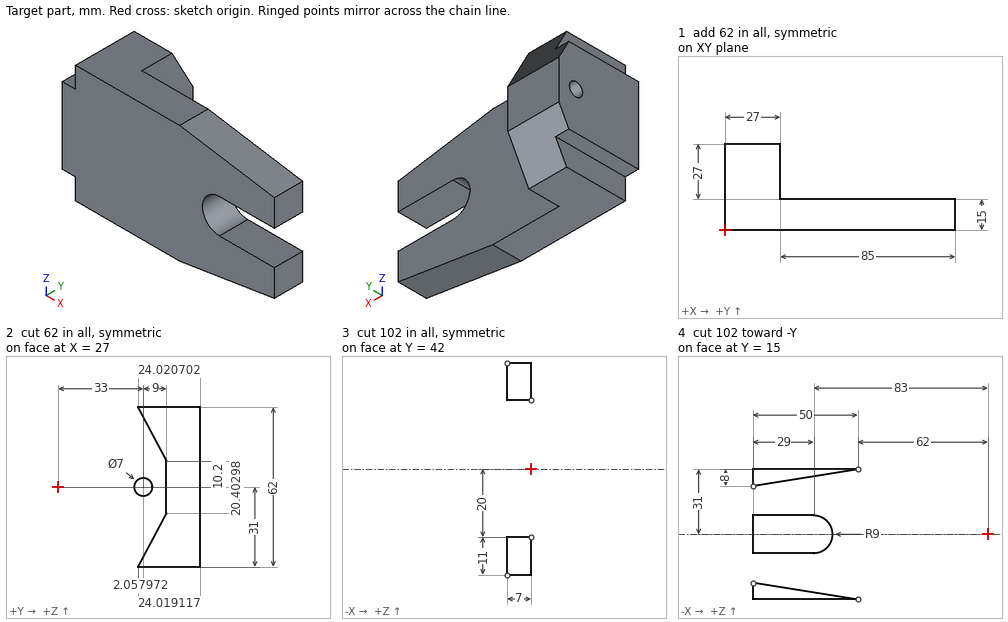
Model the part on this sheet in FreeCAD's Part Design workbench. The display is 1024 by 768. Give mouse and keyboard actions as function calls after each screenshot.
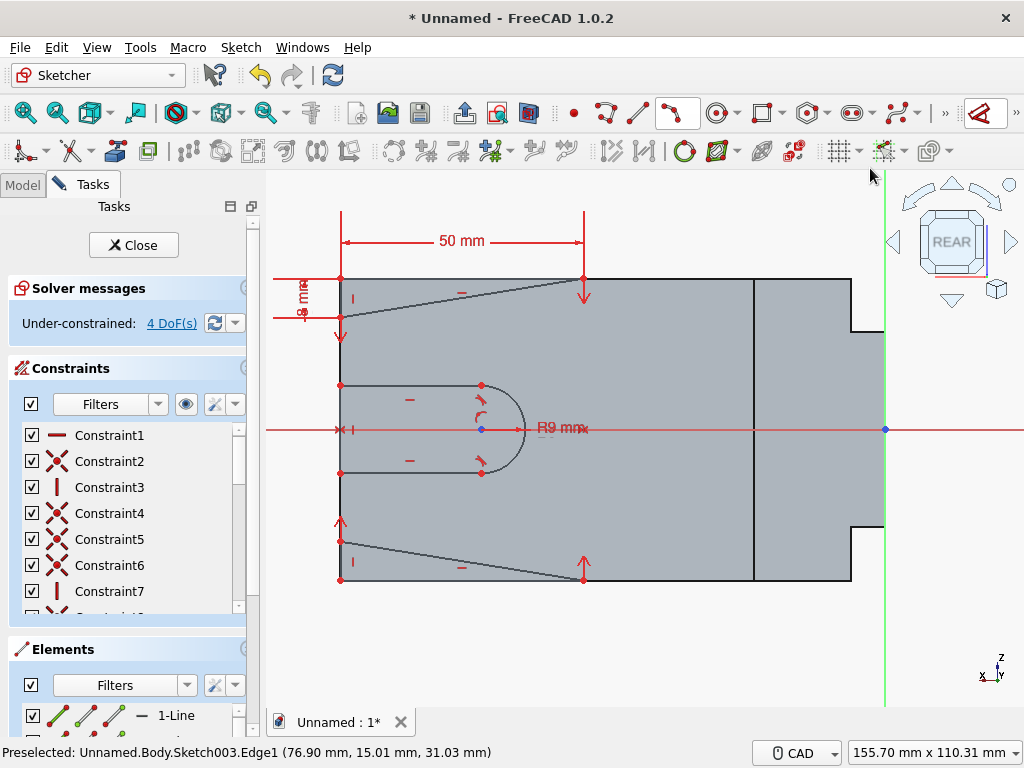
click(439, 386)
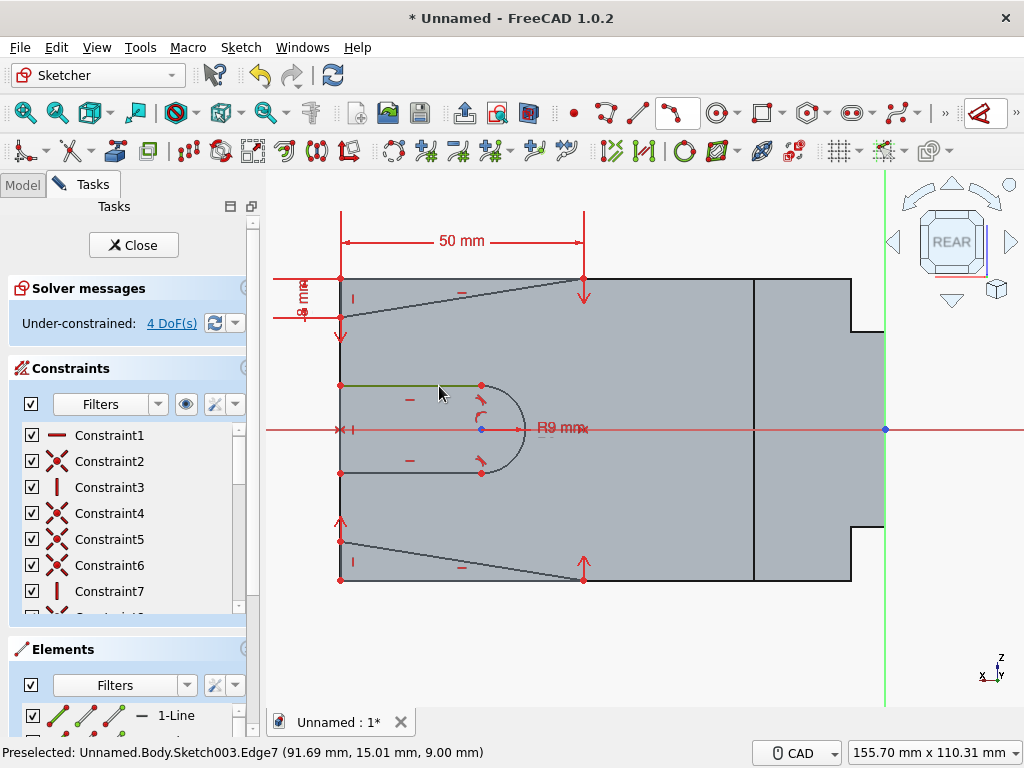
click(1002, 114)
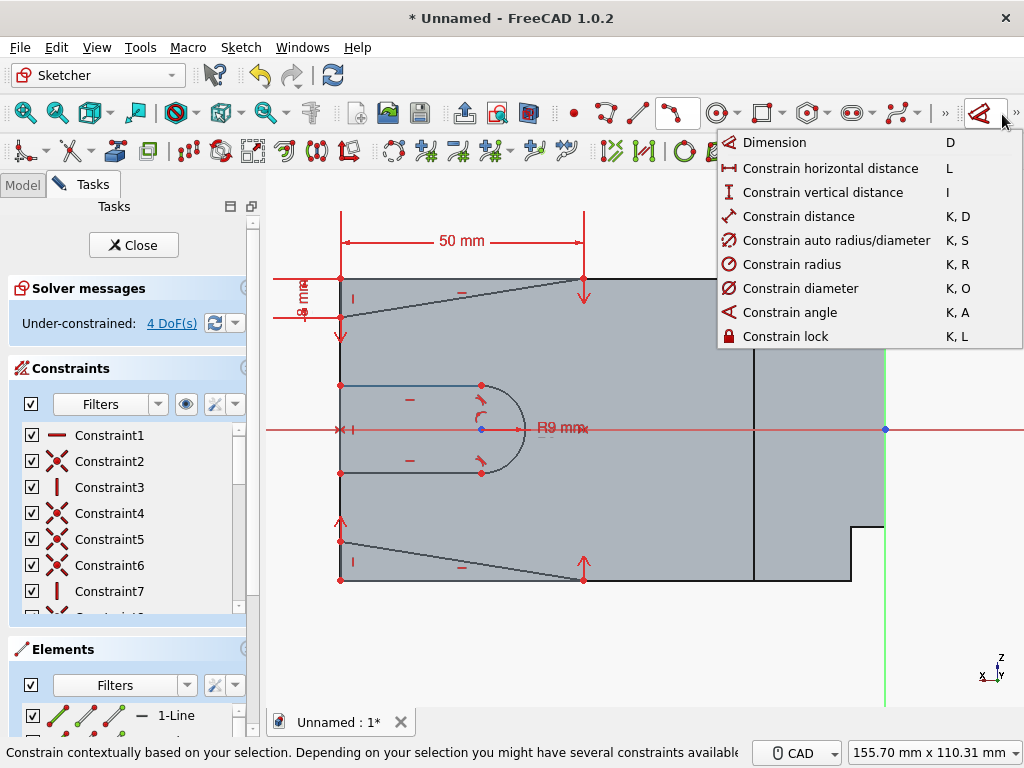
click(870, 168)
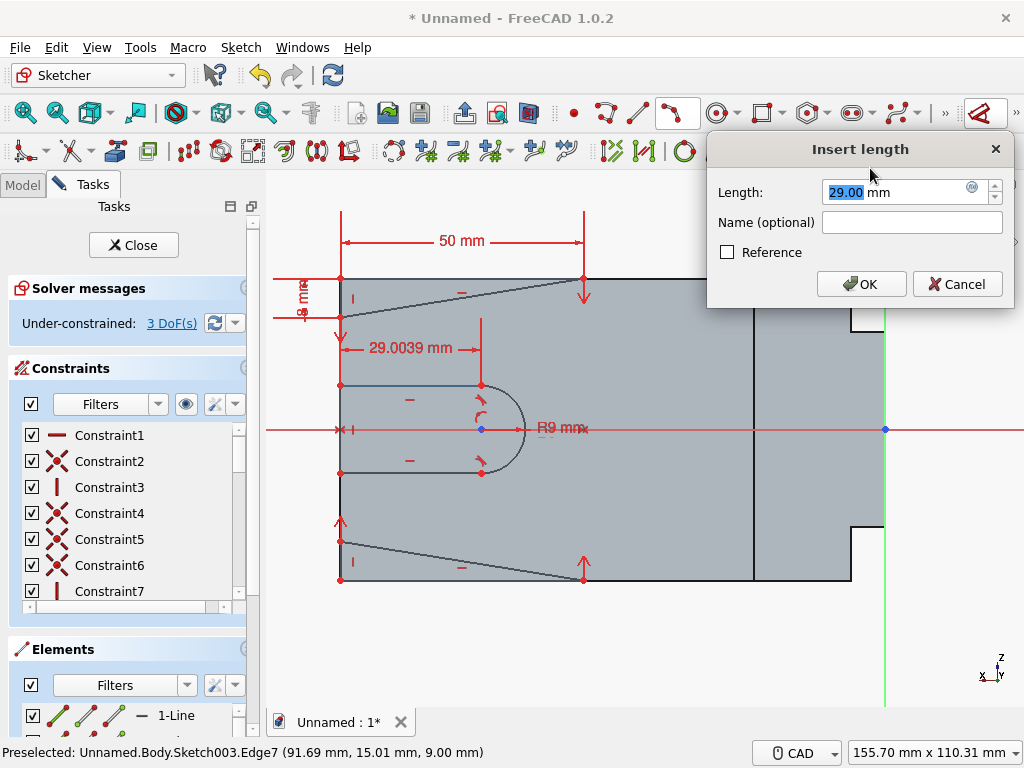
text(29)
key(Return)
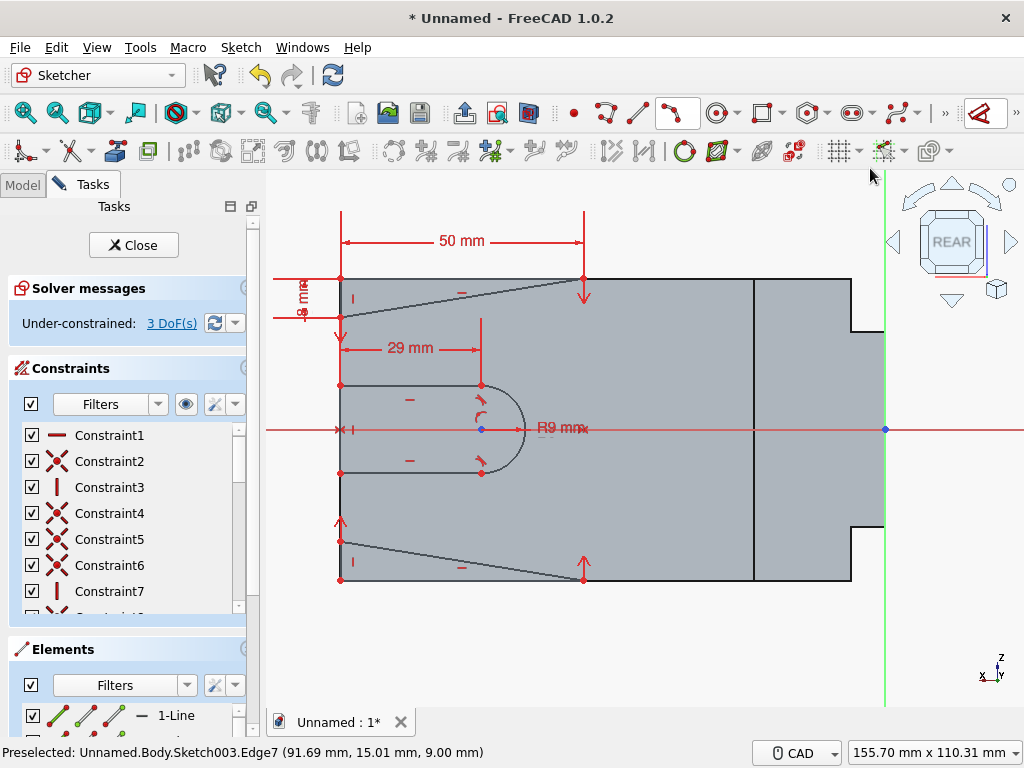
click(584, 279)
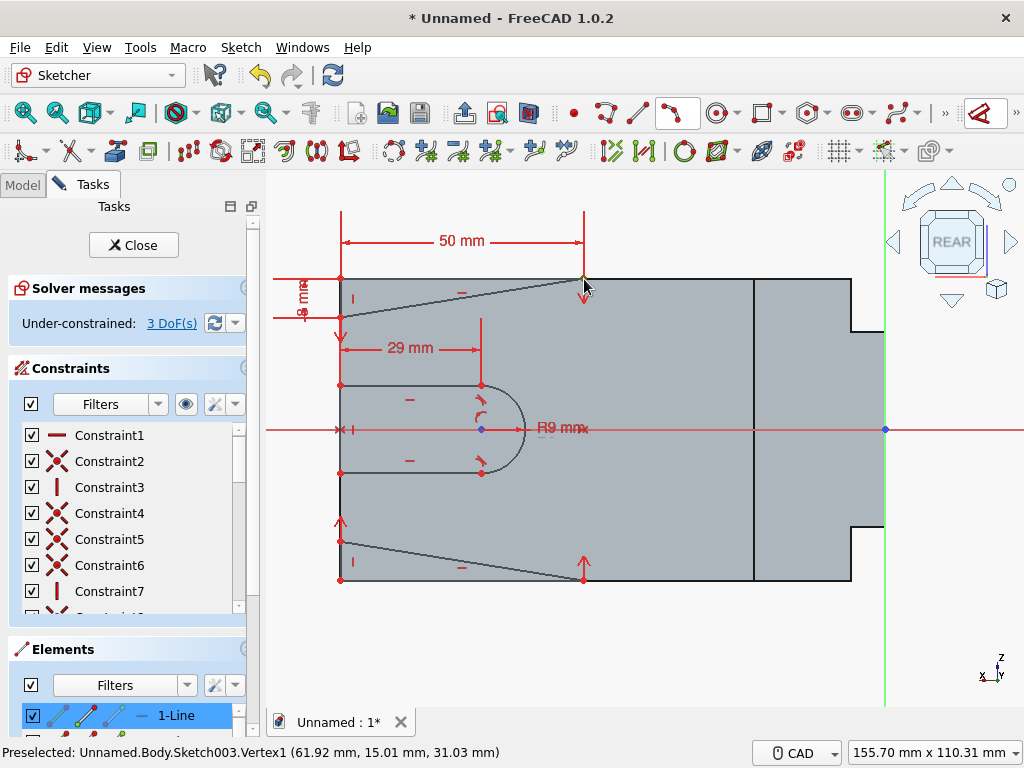
click(1002, 114)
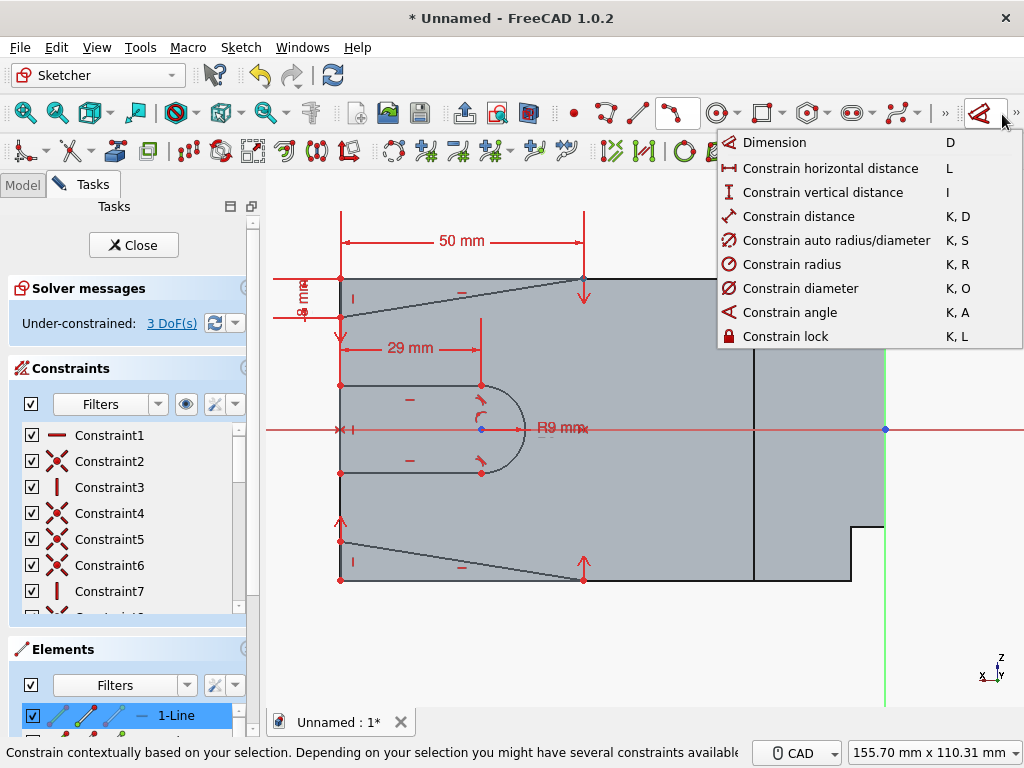
click(870, 168)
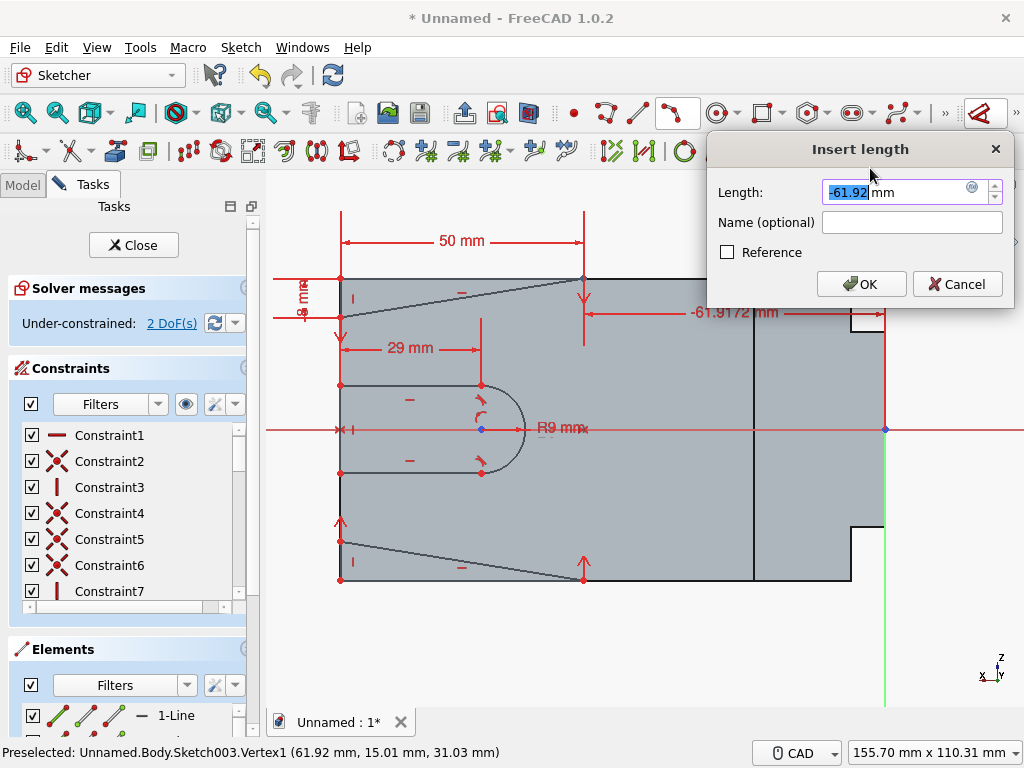
text(-62)
key(Return)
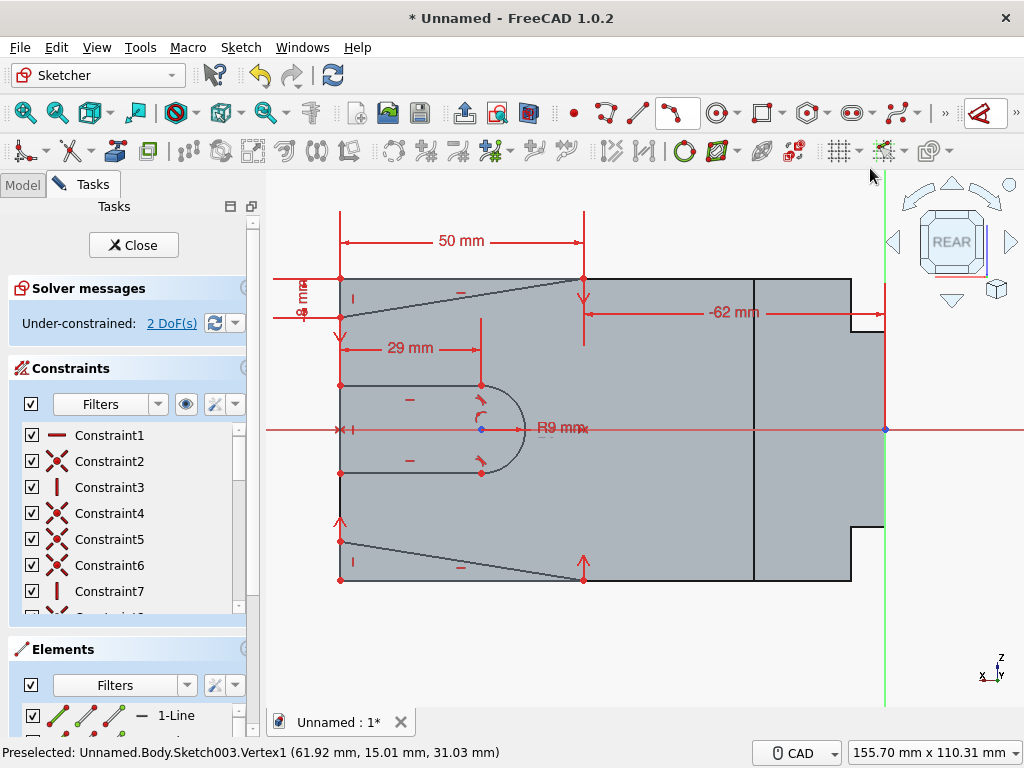
click(584, 279)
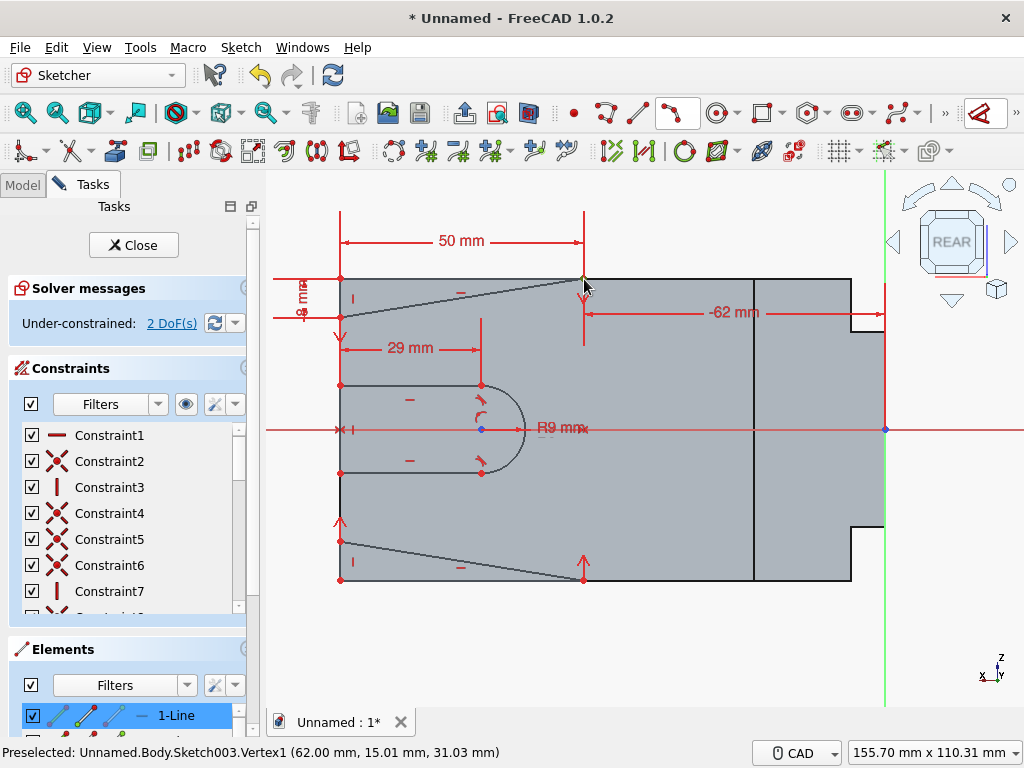
click(1002, 114)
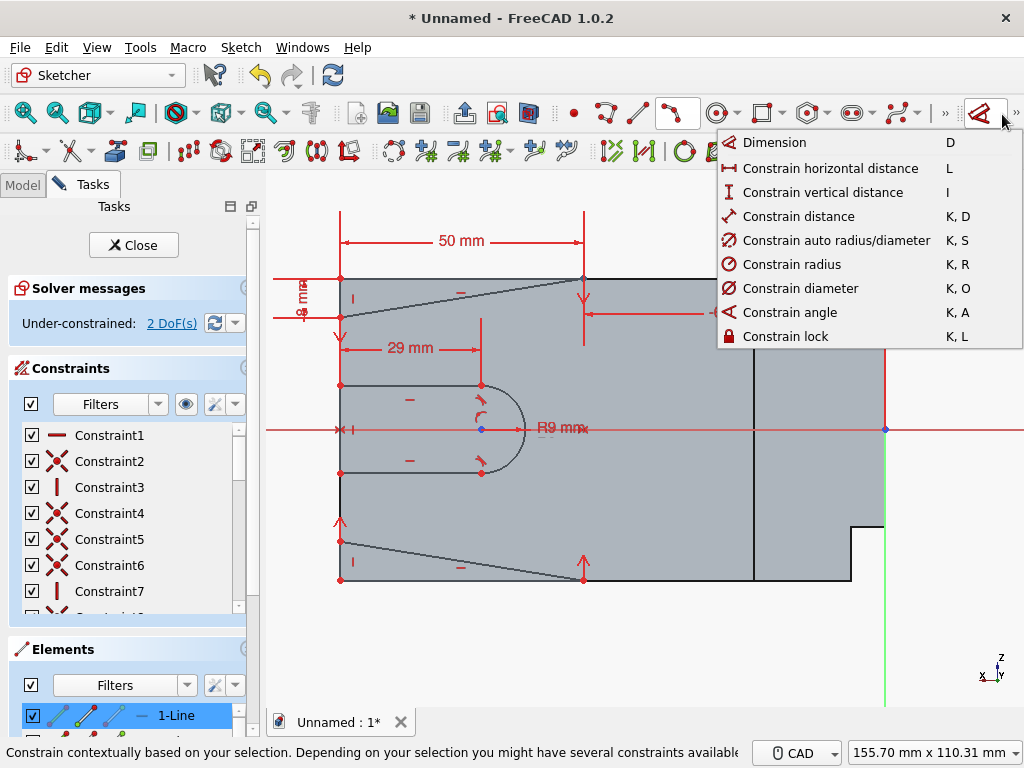
click(870, 192)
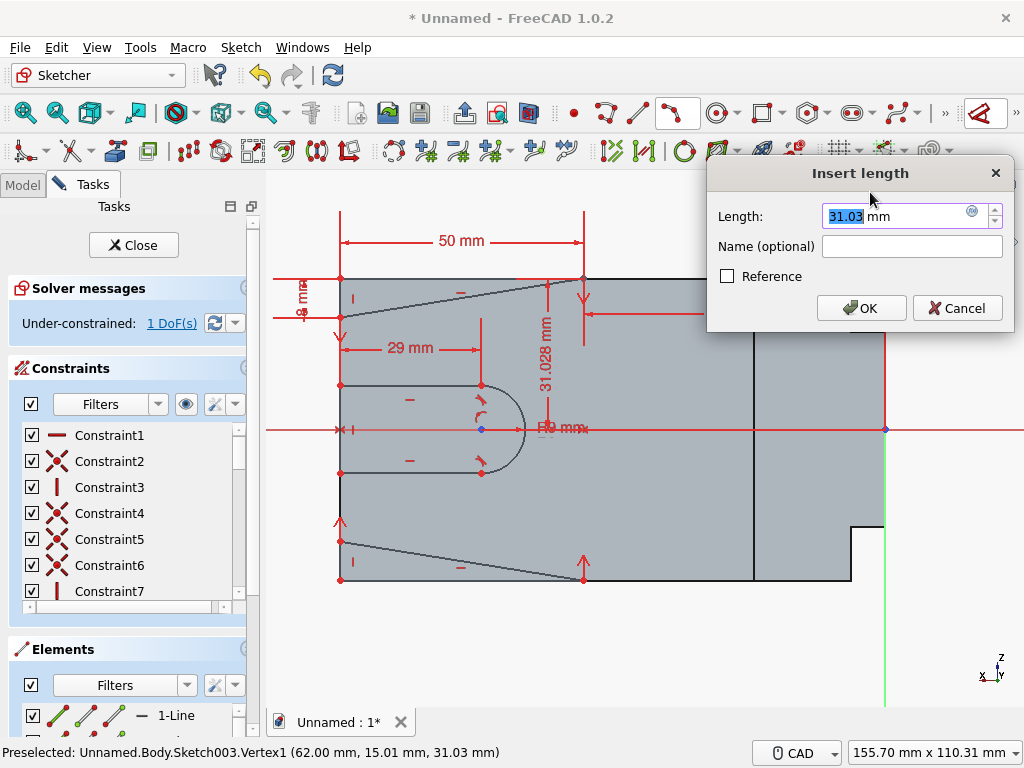
text(31)
key(Return)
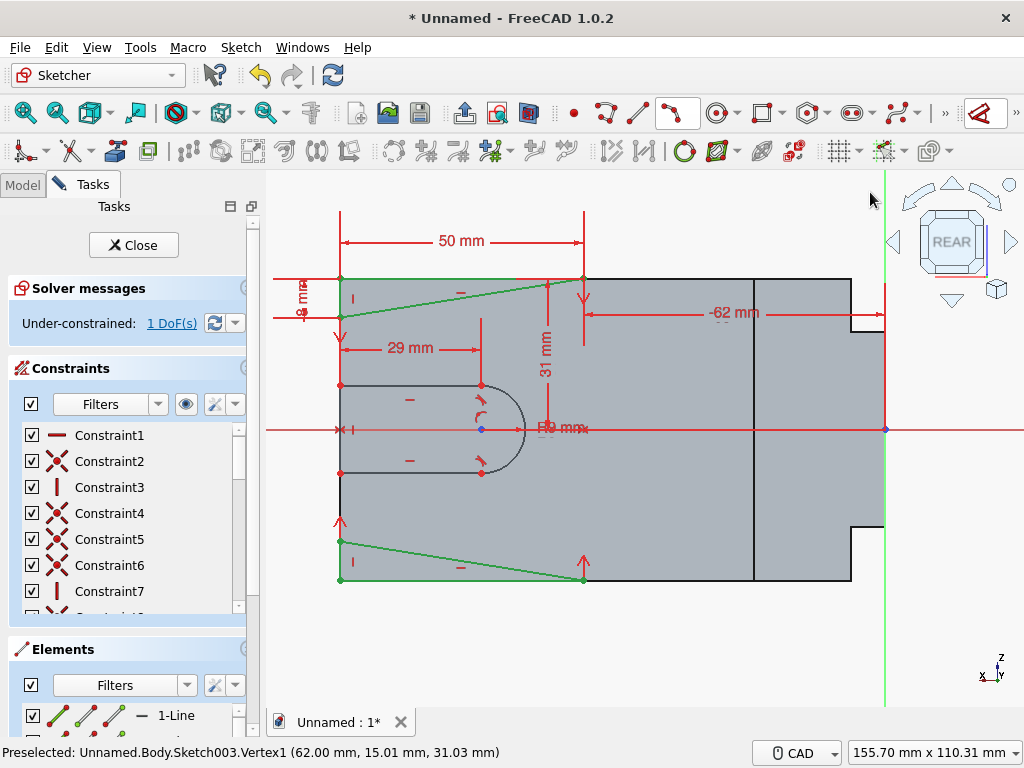
click(481, 386)